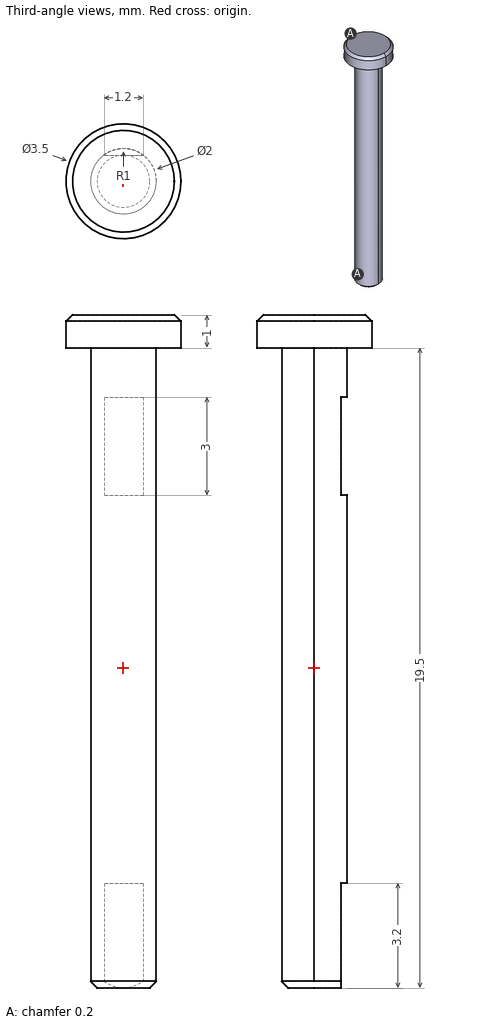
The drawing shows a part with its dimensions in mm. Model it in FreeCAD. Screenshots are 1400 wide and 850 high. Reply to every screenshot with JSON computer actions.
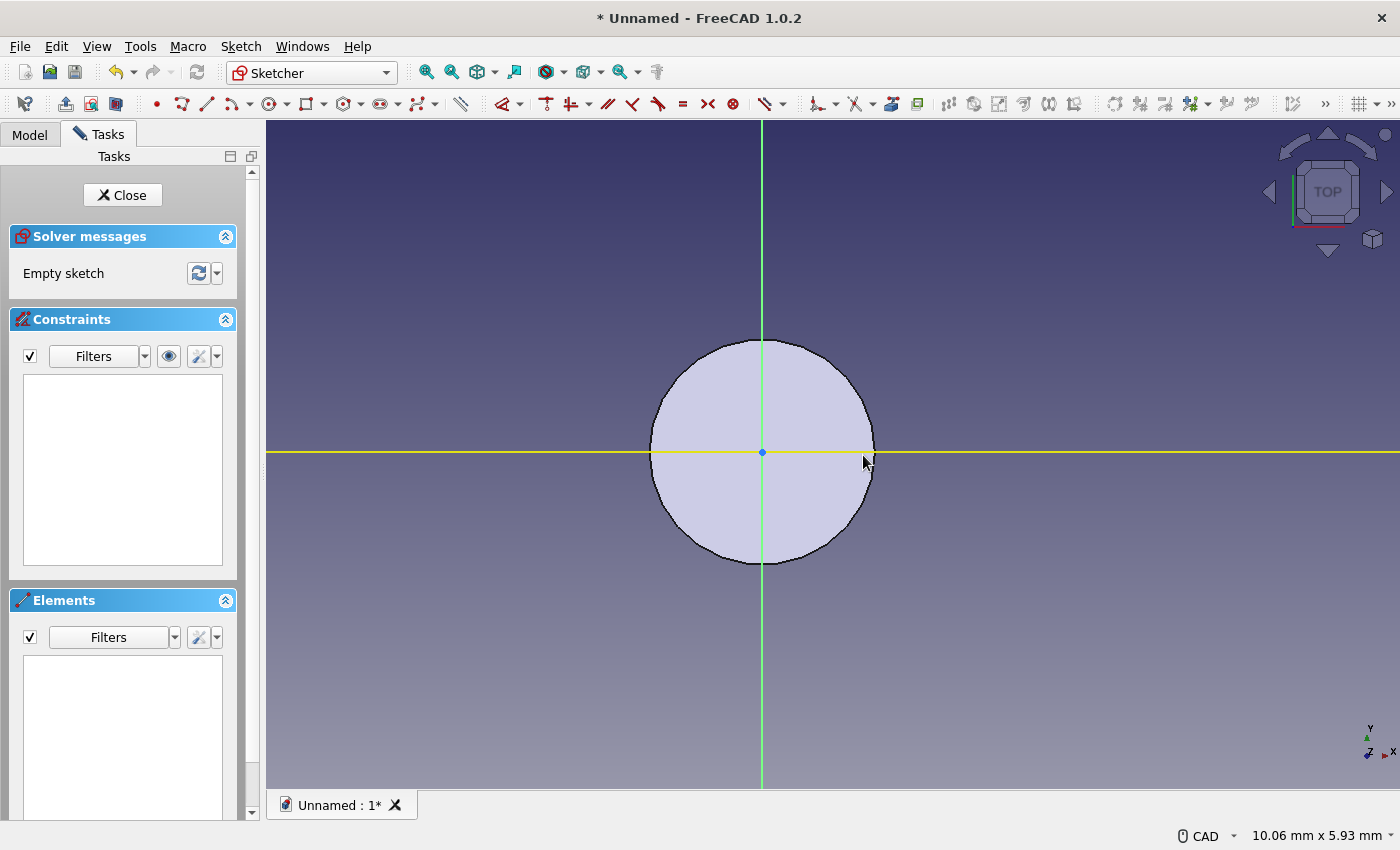
{"action": "key", "text": "g c"}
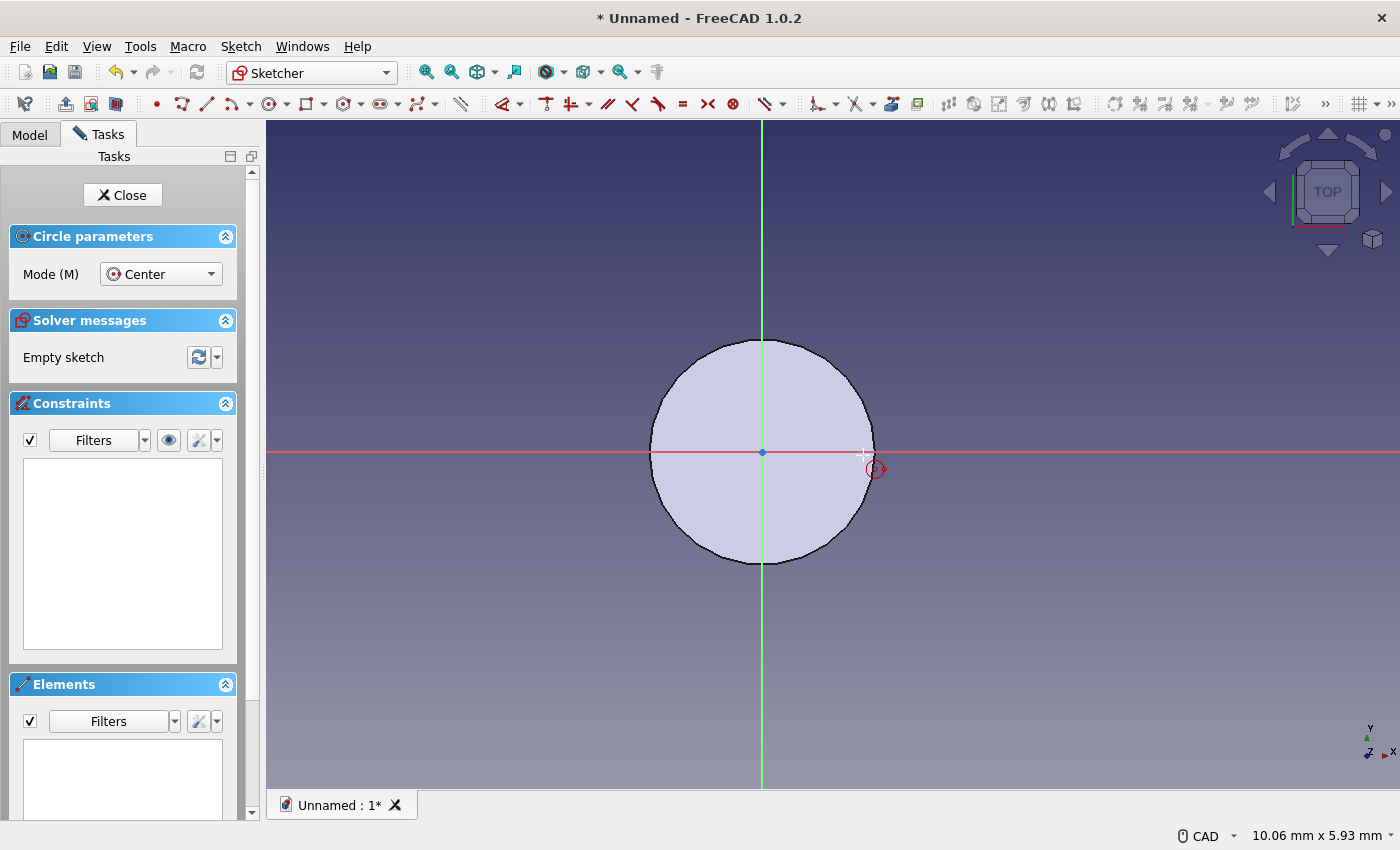
{"action": "left_click", "coordinate": [762, 452]}
{"action": "mouse_move", "coordinate": [902, 313]}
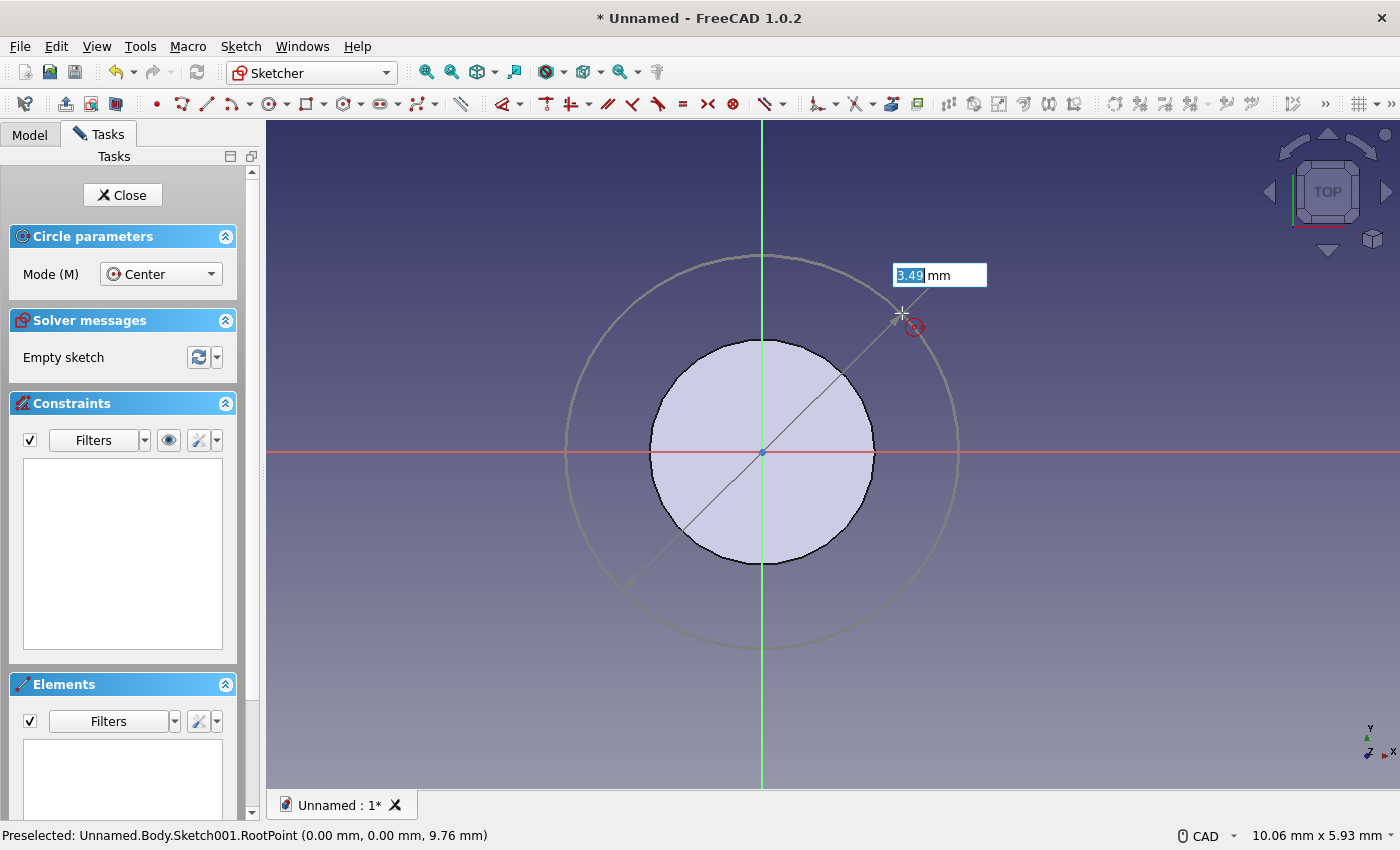
{"action": "type", "text": "3.5"}
{"action": "key", "text": "Return"}
{"action": "key", "text": "Escape"}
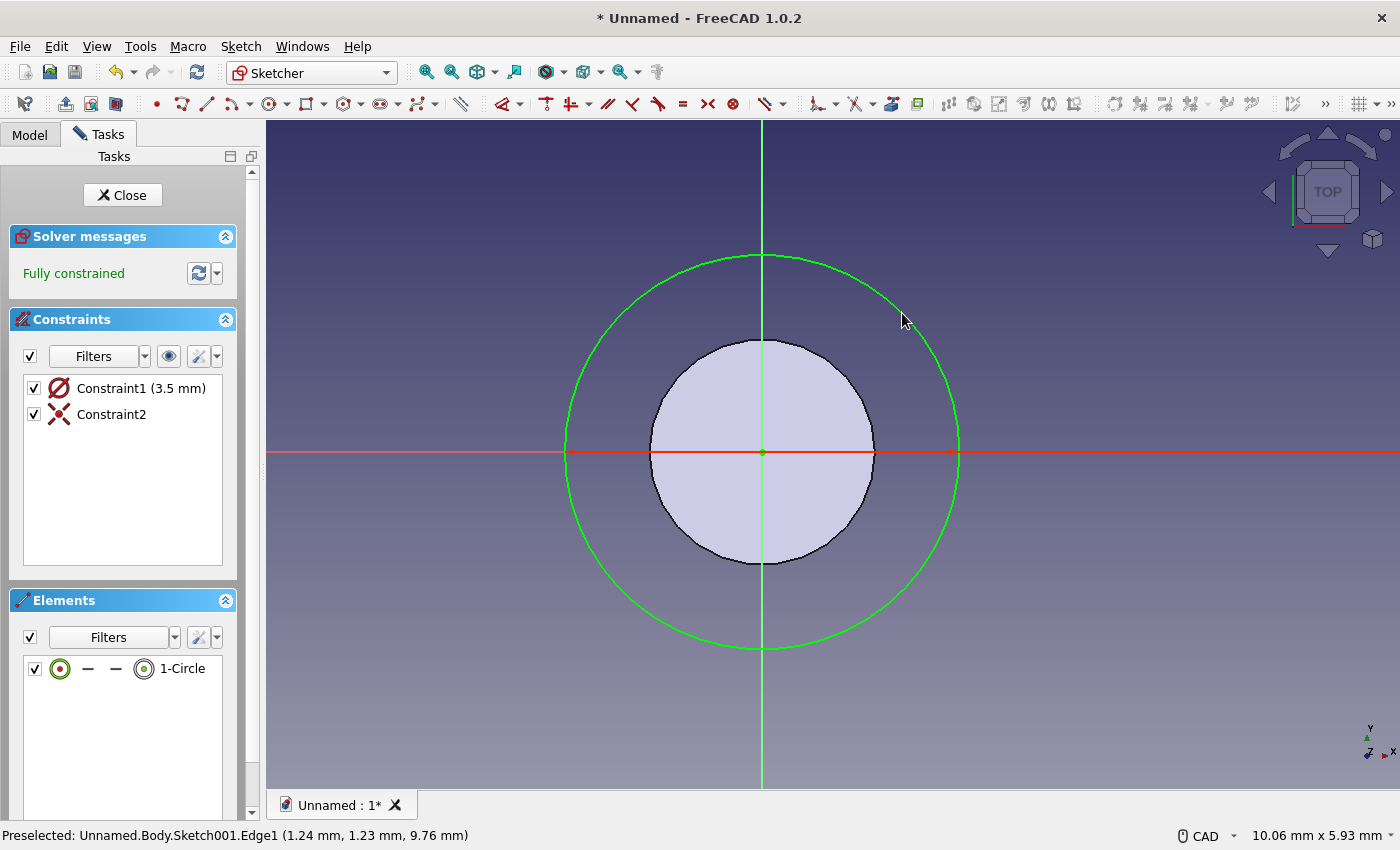
{"action": "left_click", "coordinate": [123, 195]}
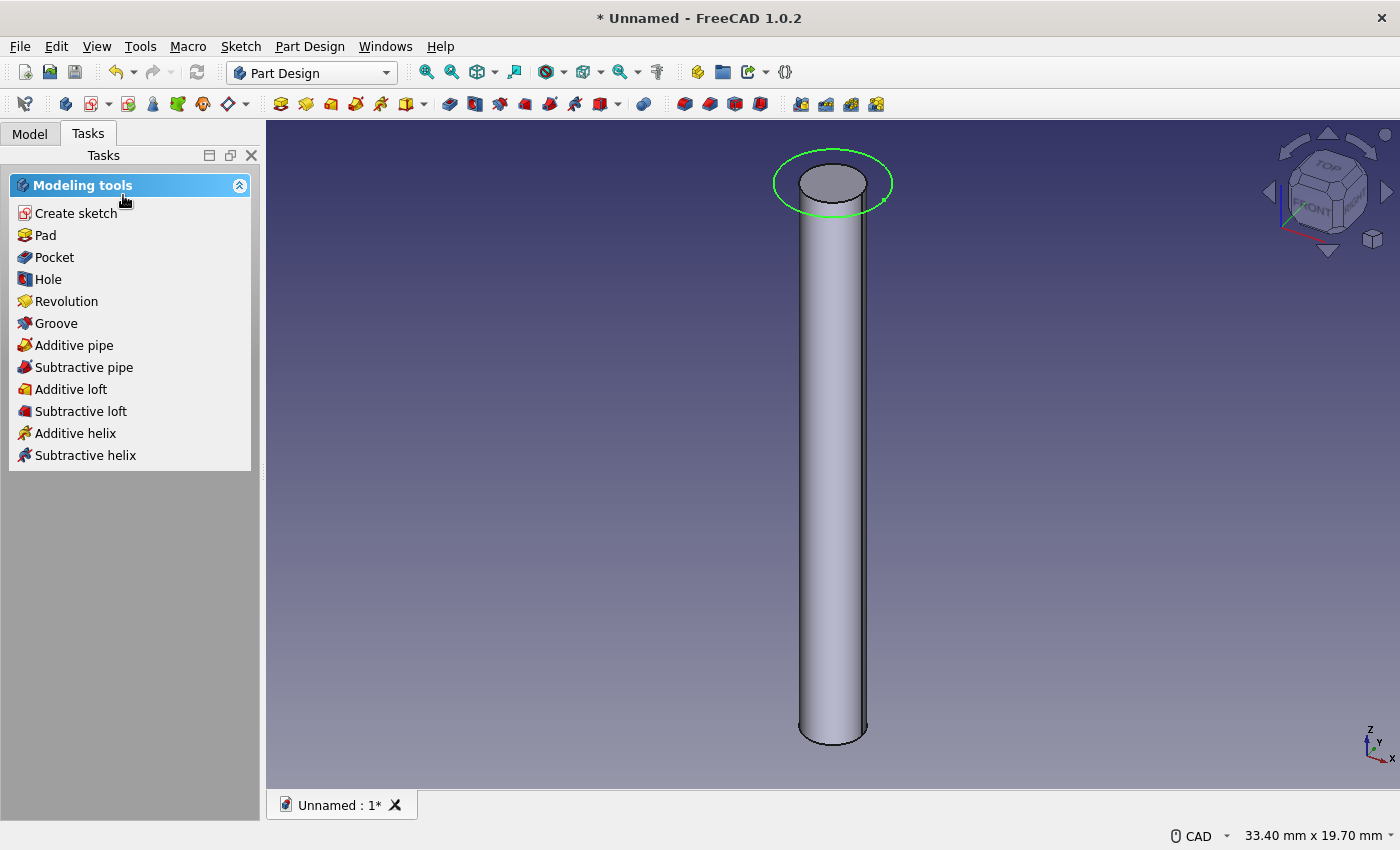
{"action": "left_click", "coordinate": [281, 104]}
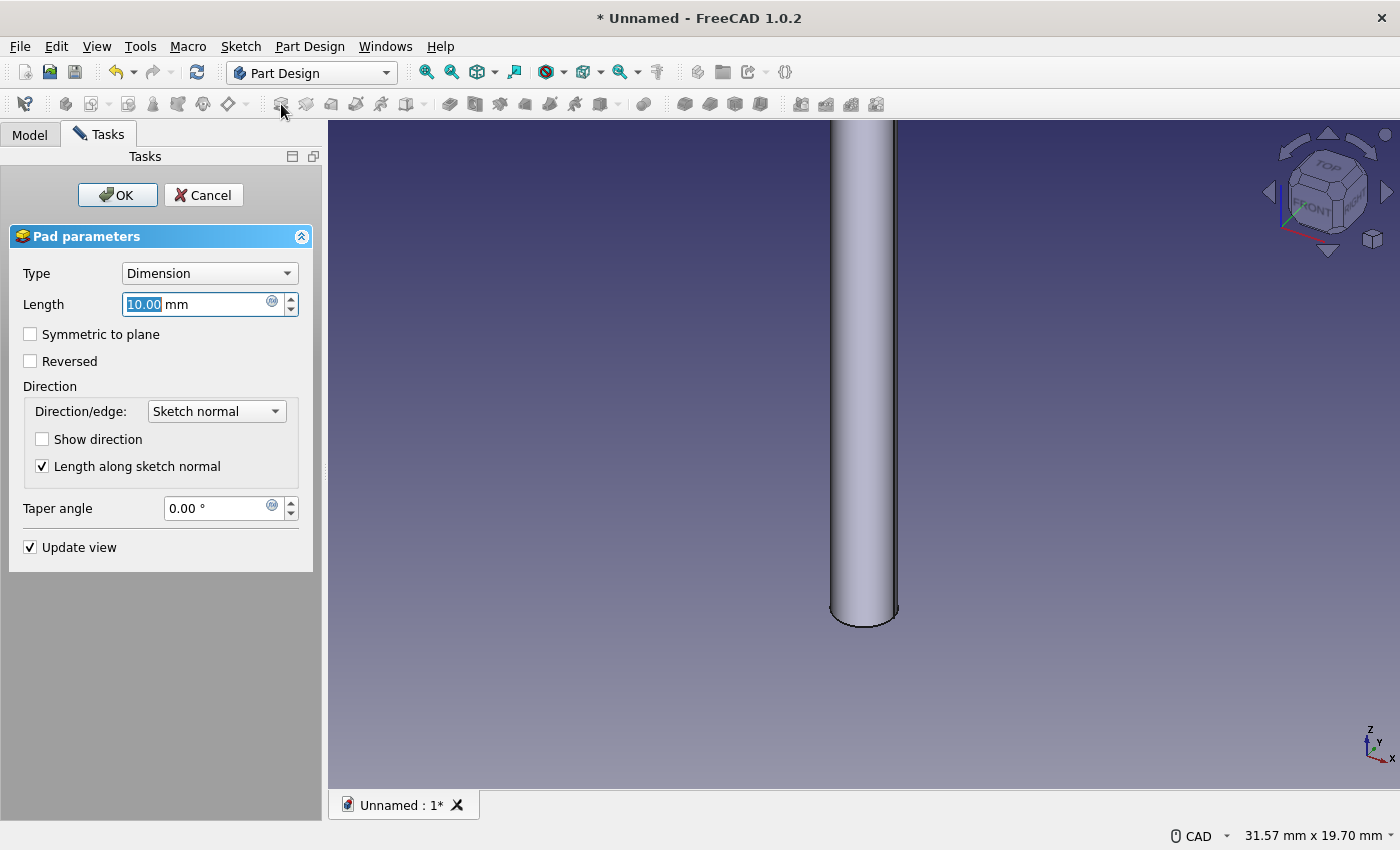
{"action": "type", "text": "1"}
{"action": "key", "text": "Tab"}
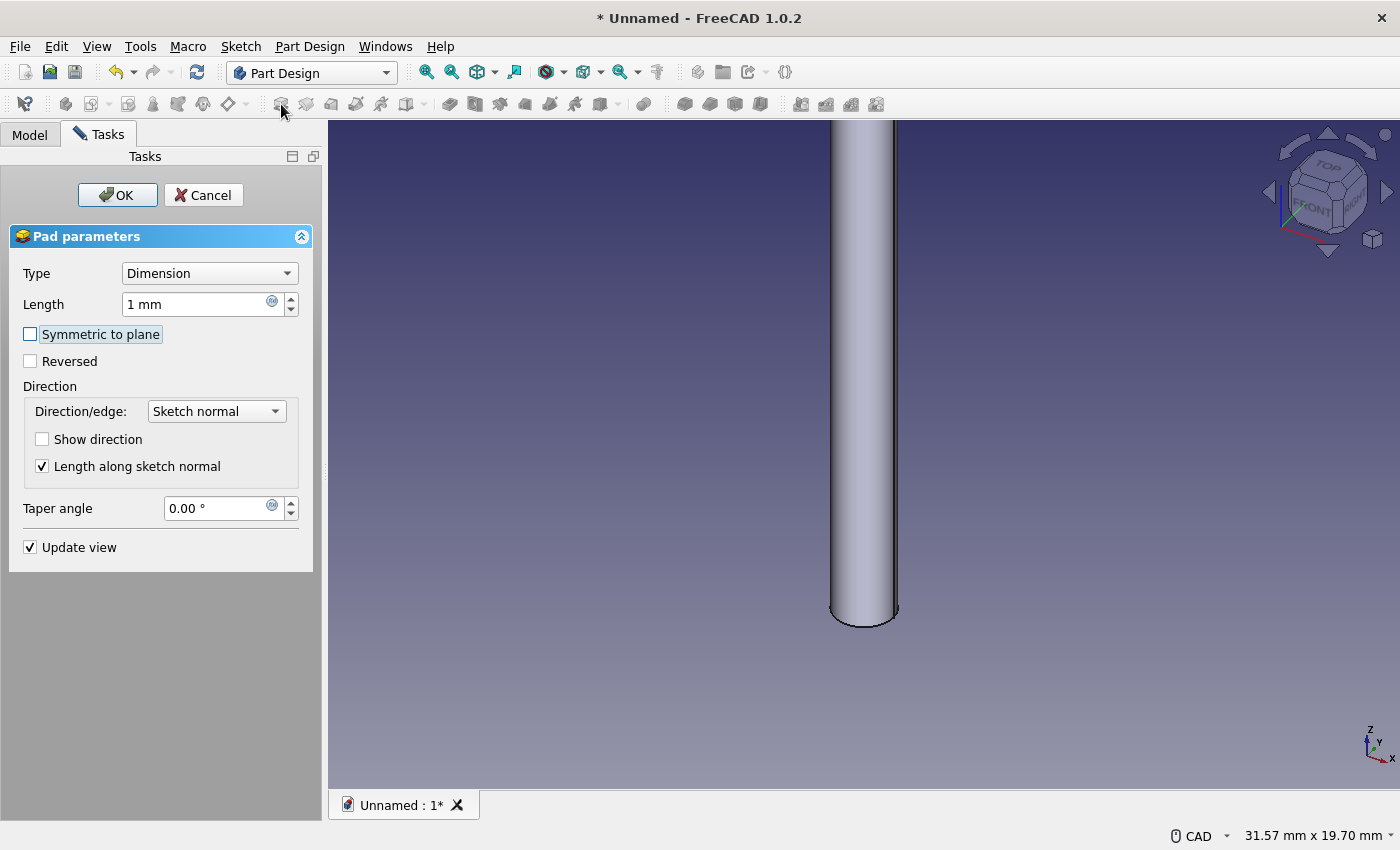
{"action": "left_click", "coordinate": [118, 195]}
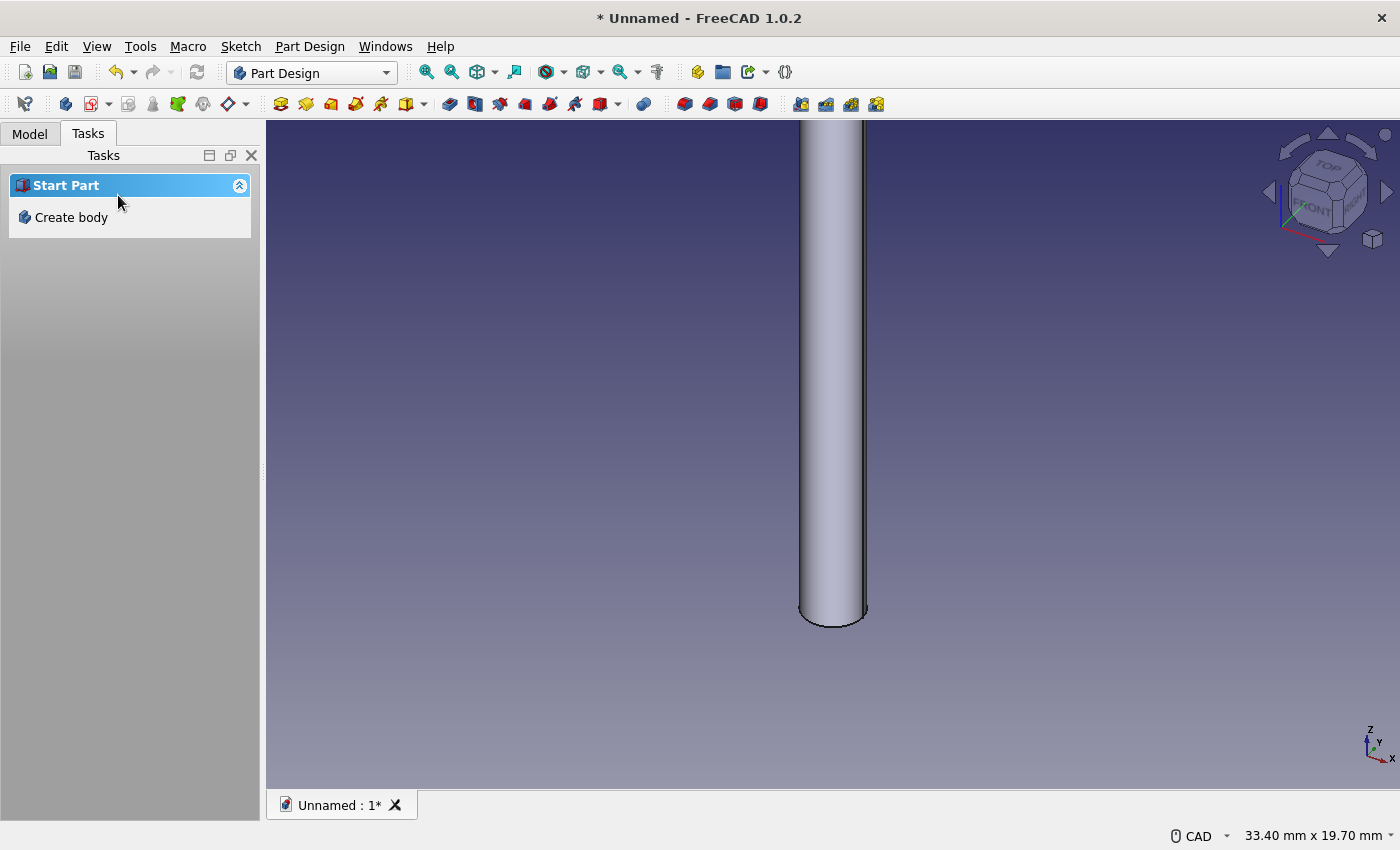
{"action": "key", "text": "v f"}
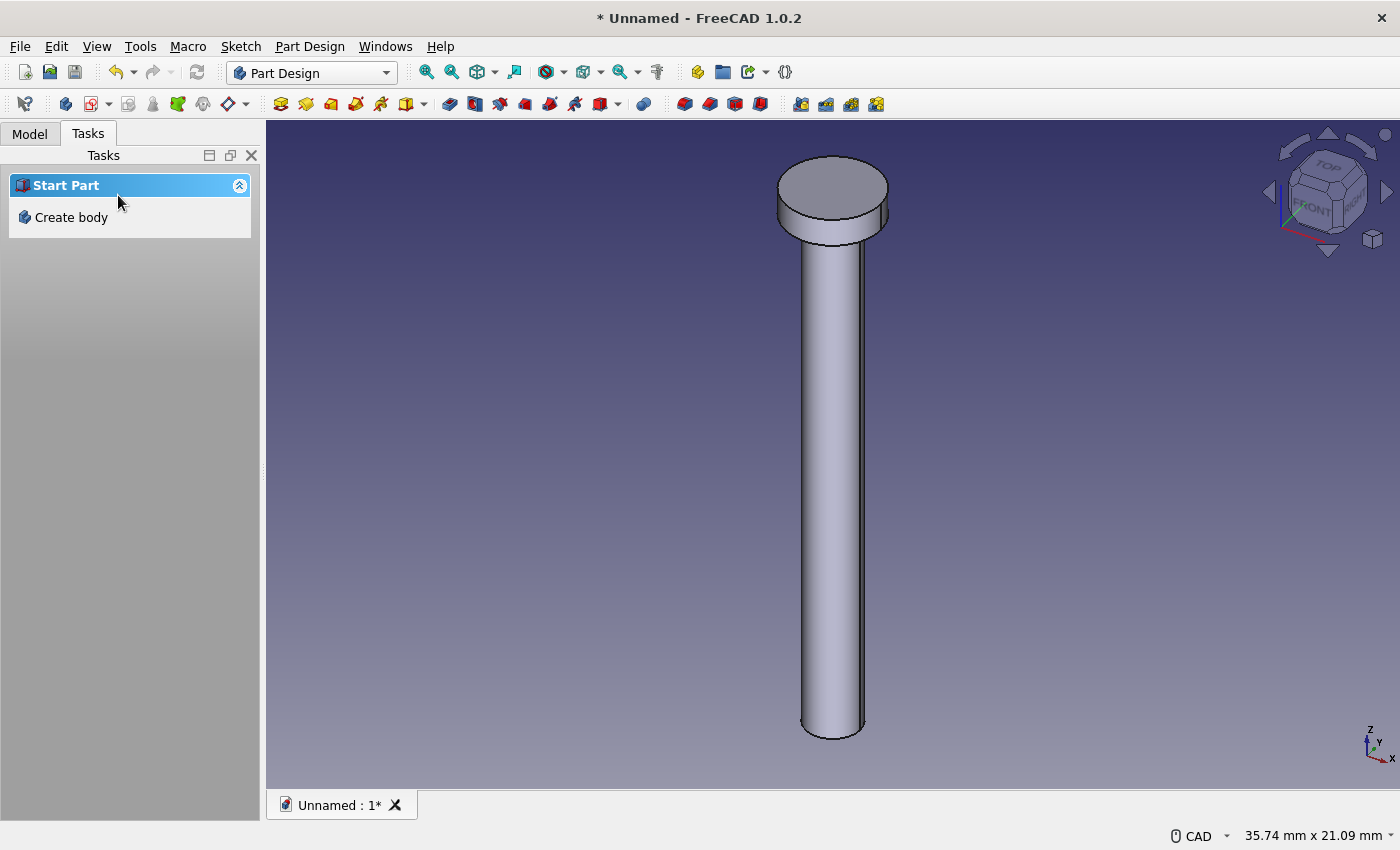
{"action": "left_click", "coordinate": [778, 190]}